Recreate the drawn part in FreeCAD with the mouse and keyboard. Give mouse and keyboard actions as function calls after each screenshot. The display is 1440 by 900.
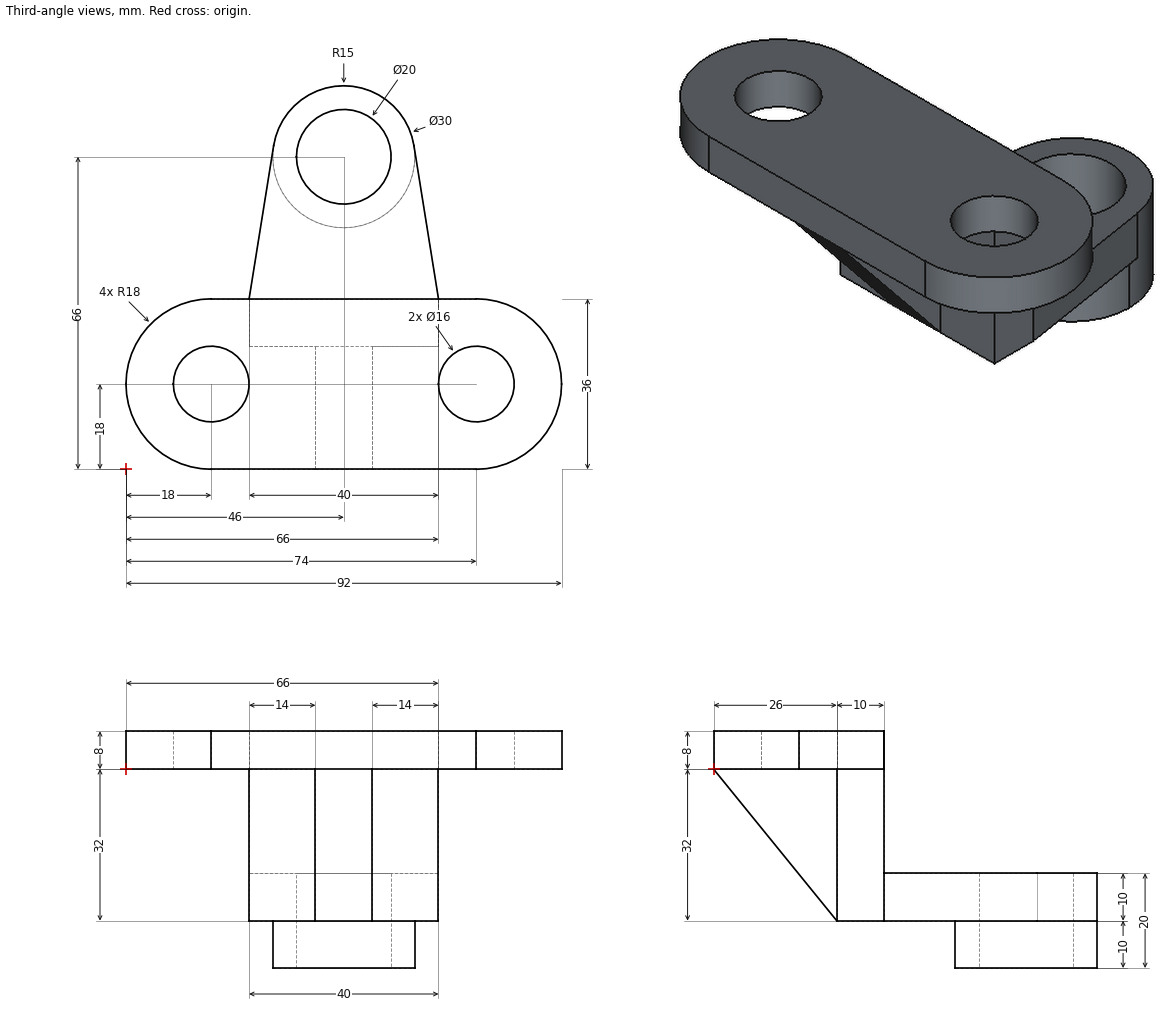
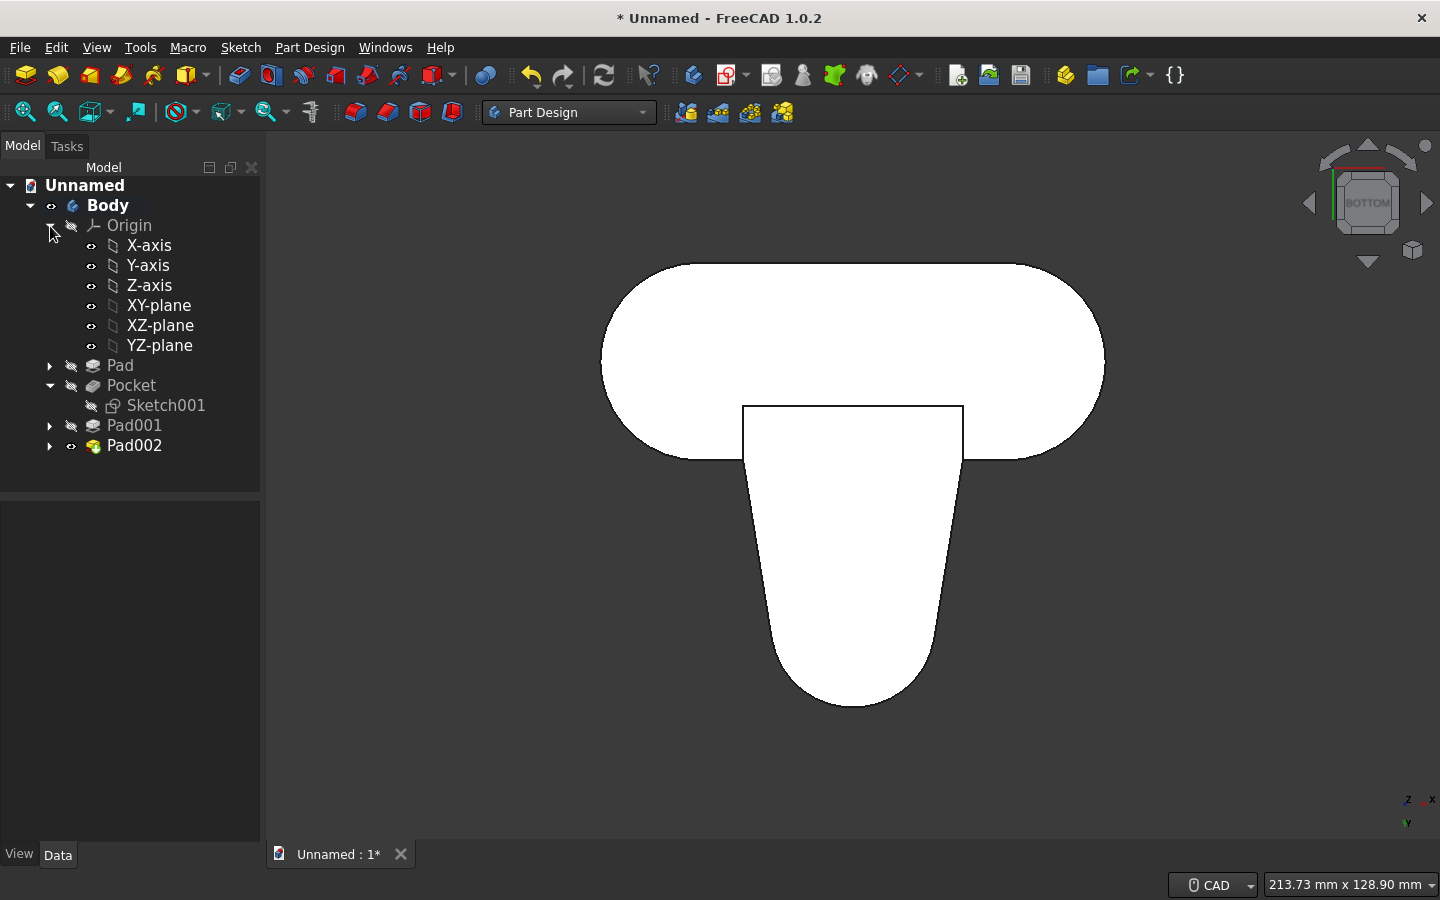
click(136, 306)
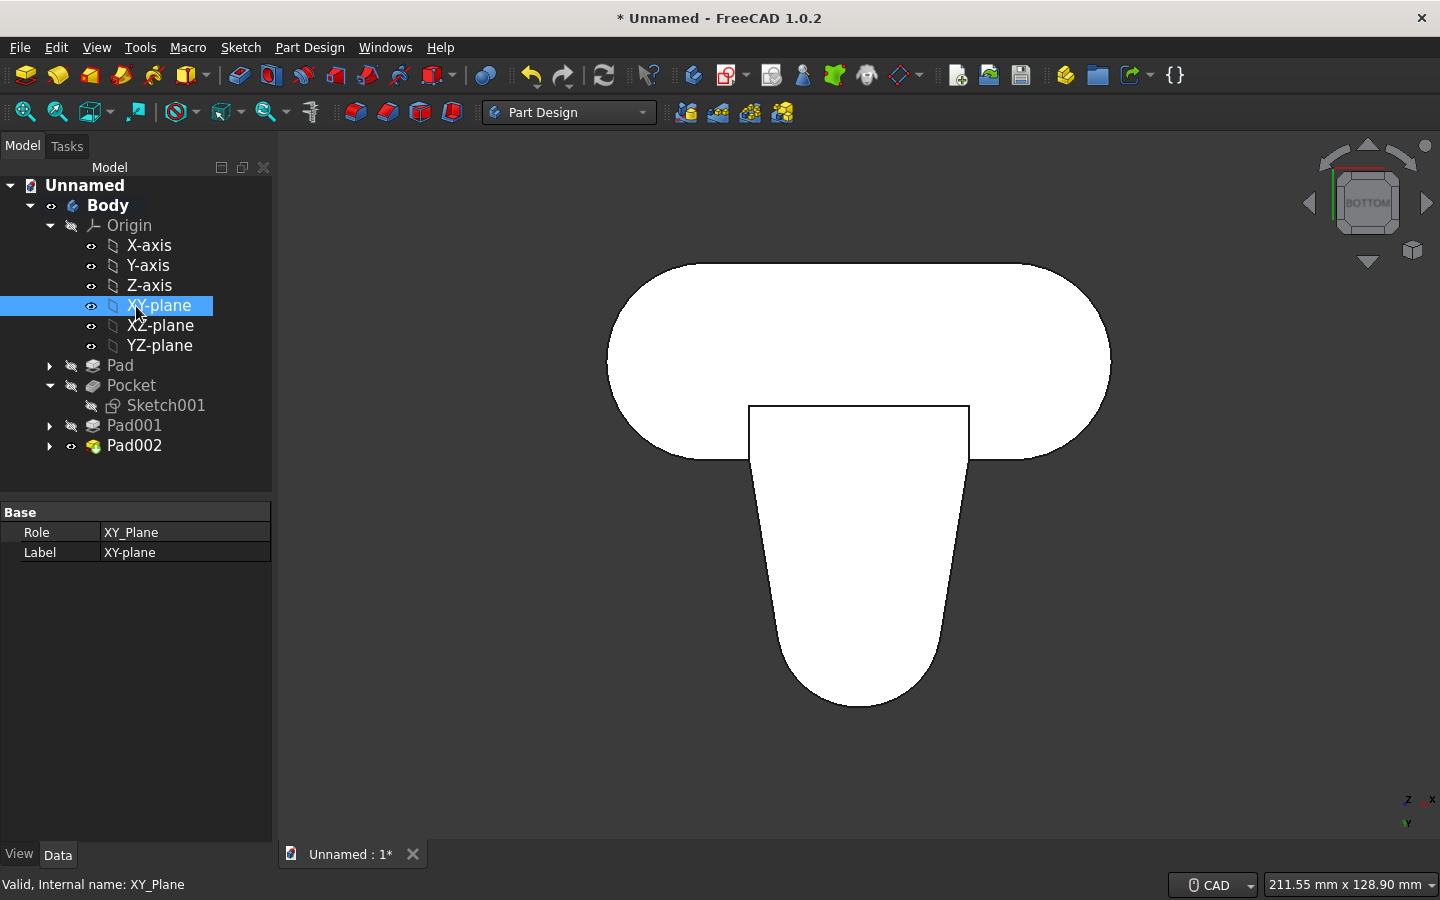
click(900, 76)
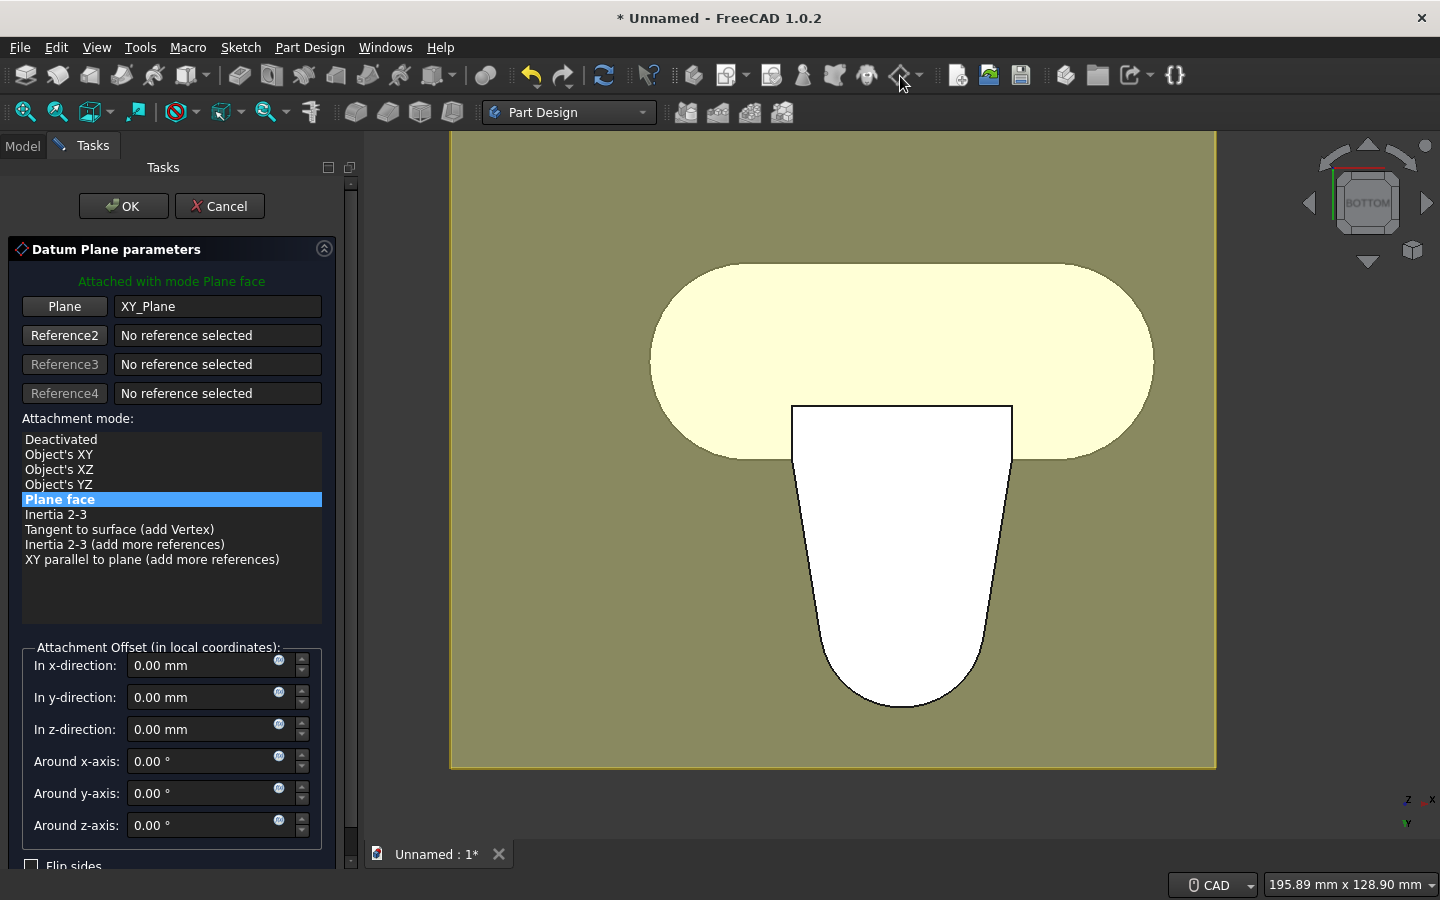
triple_click(210, 729)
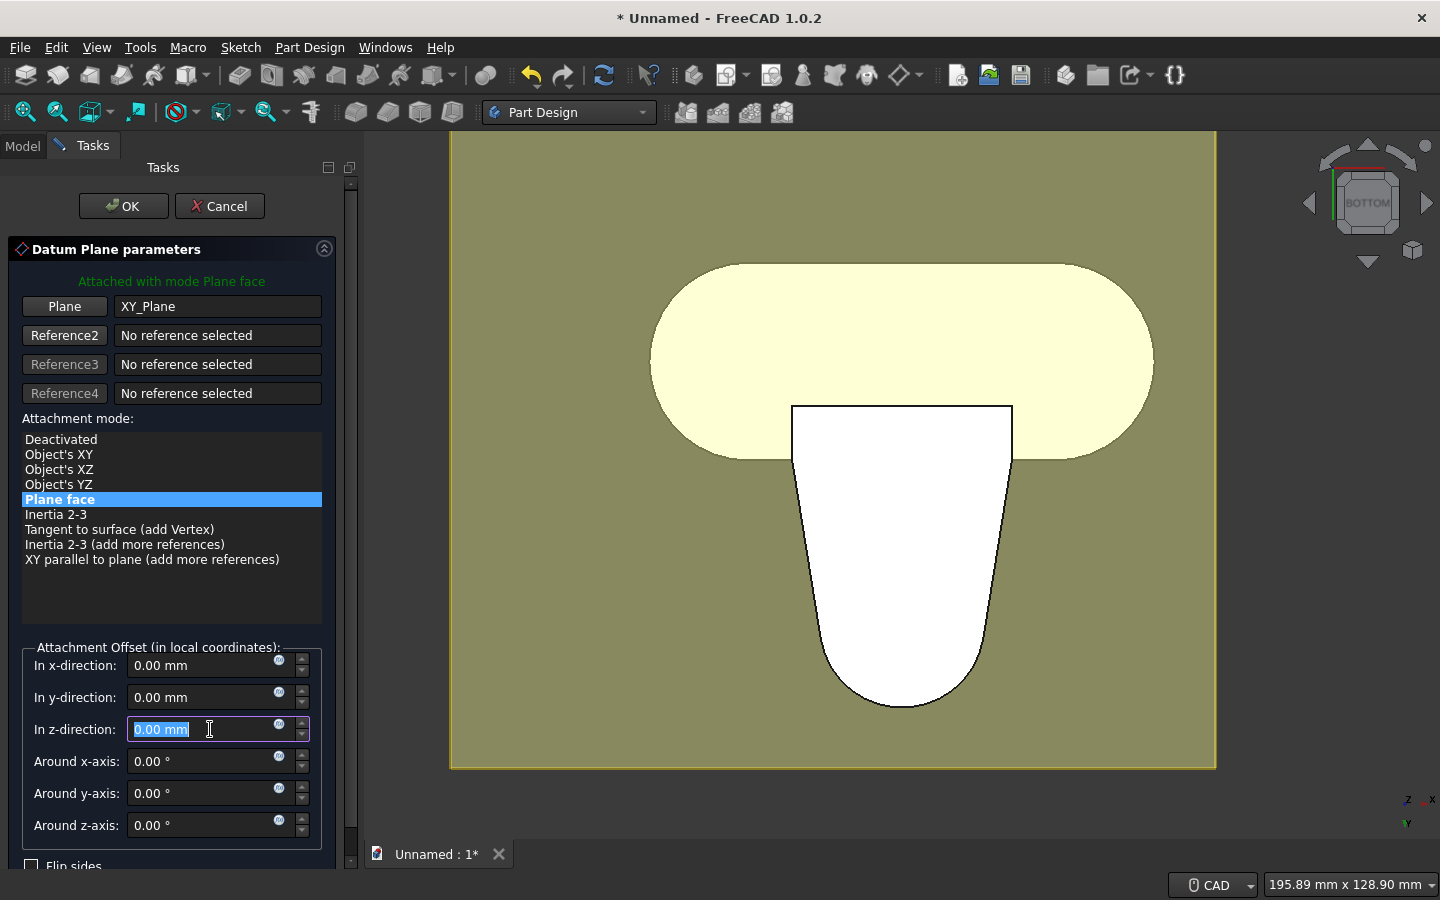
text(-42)
key(Tab)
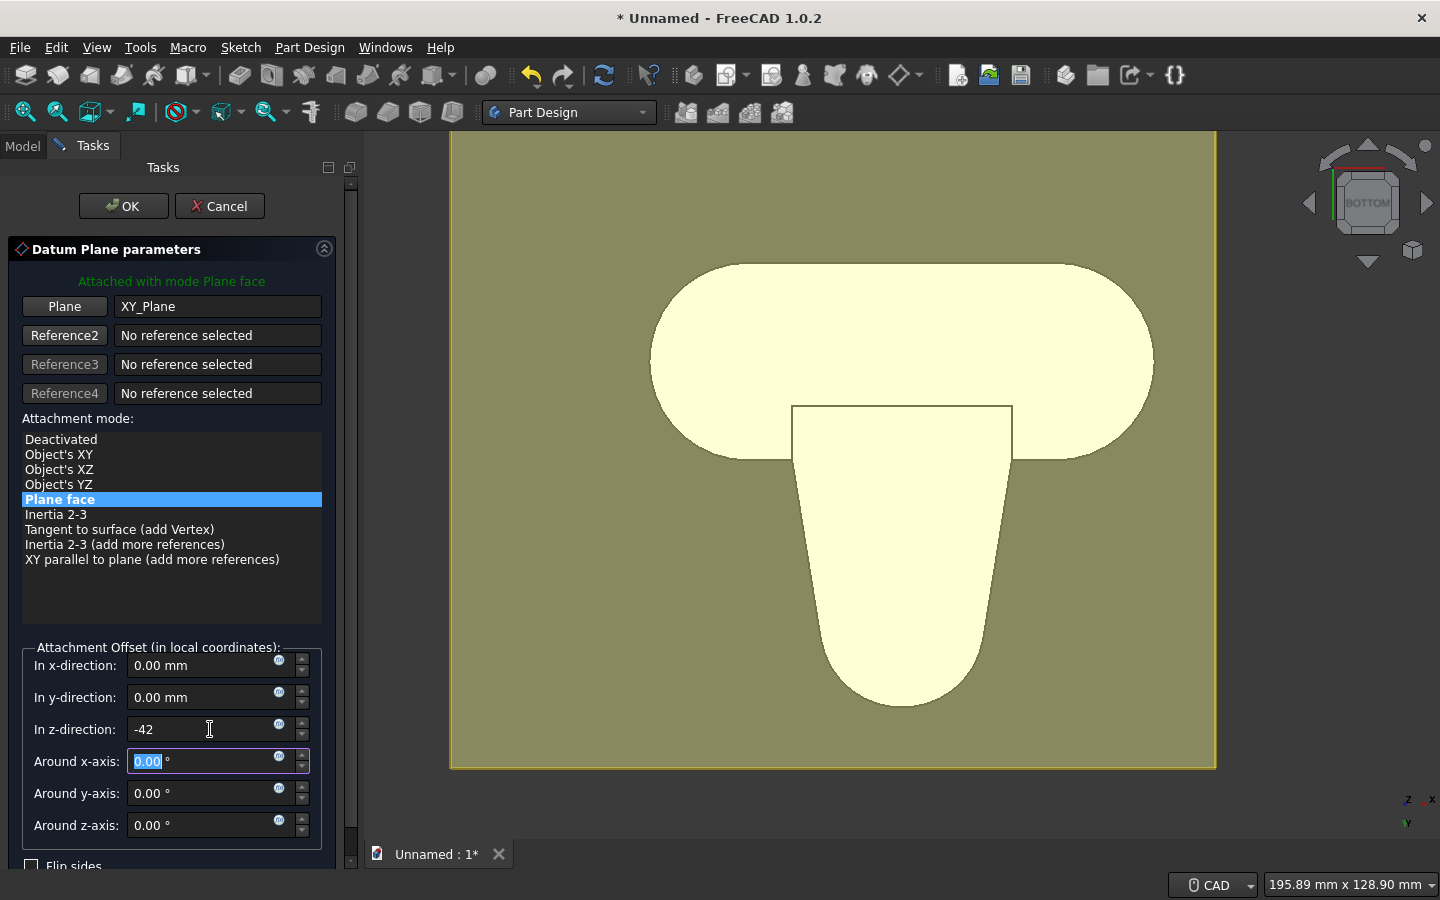
click(124, 206)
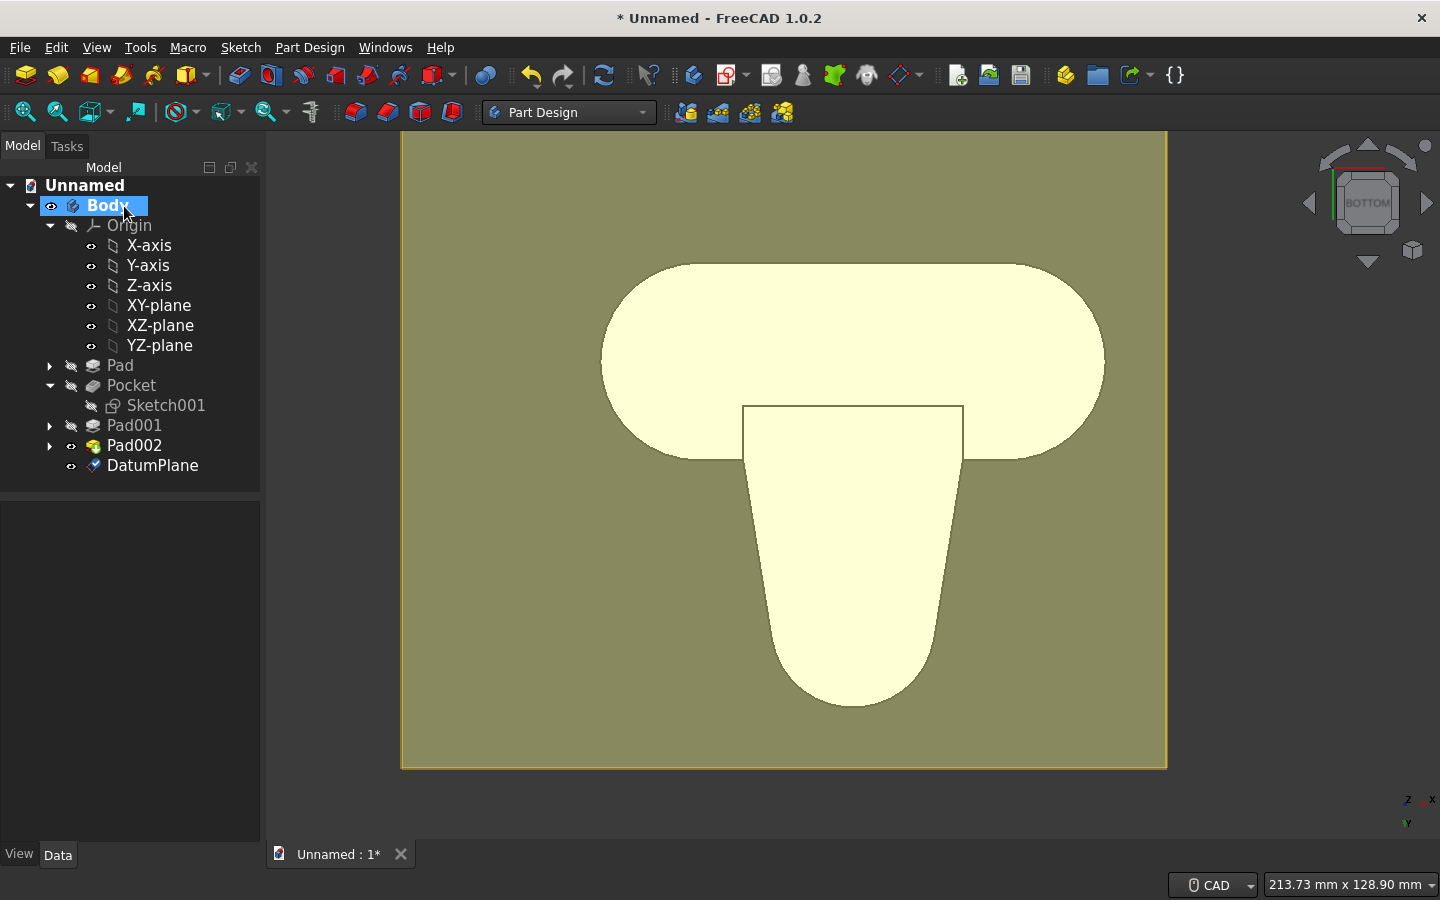
click(116, 466)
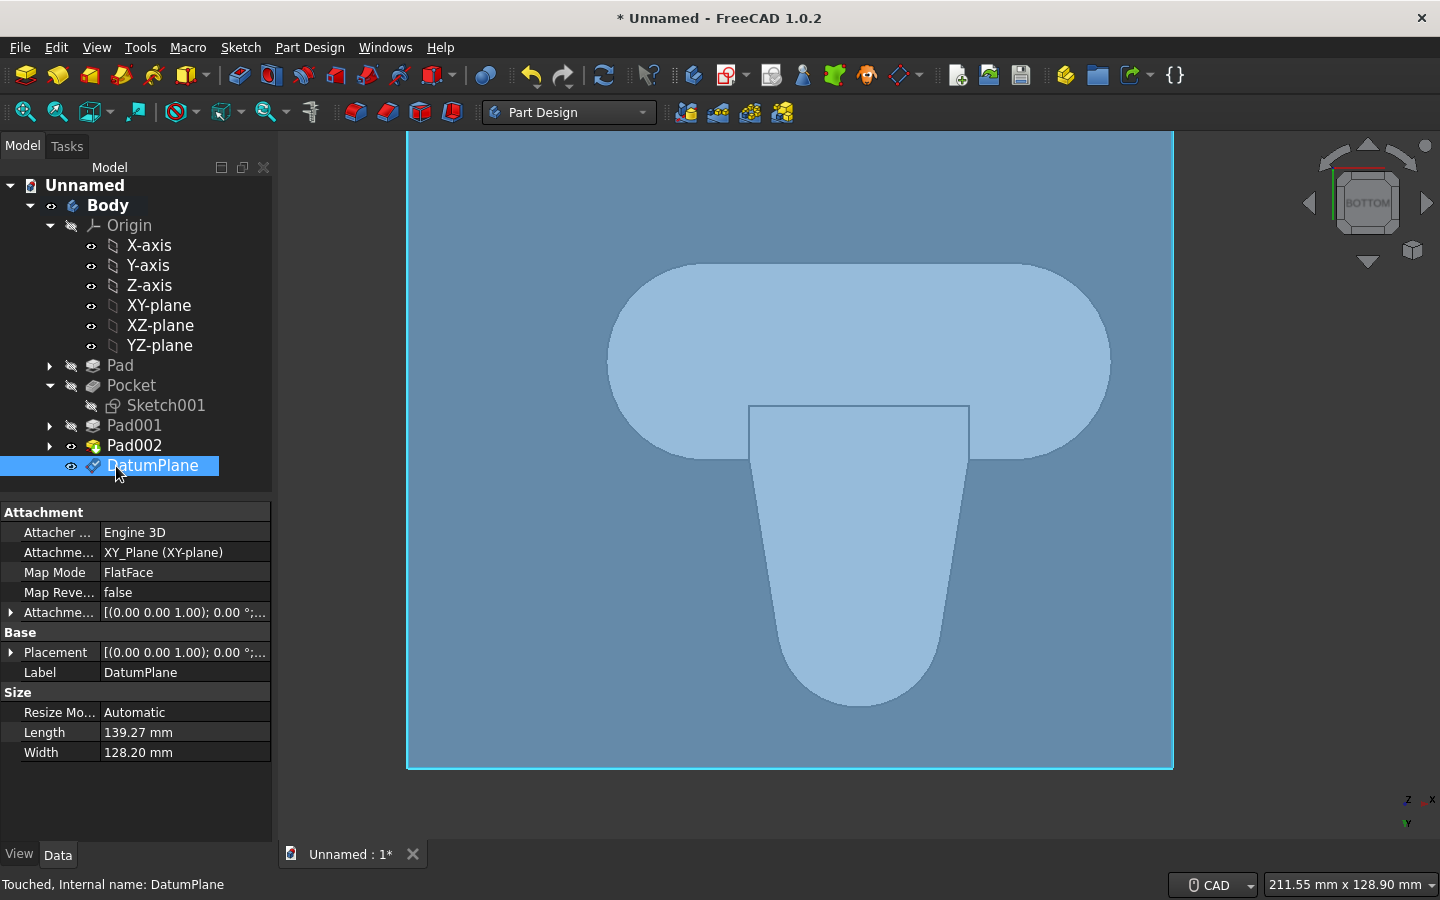
click(726, 76)